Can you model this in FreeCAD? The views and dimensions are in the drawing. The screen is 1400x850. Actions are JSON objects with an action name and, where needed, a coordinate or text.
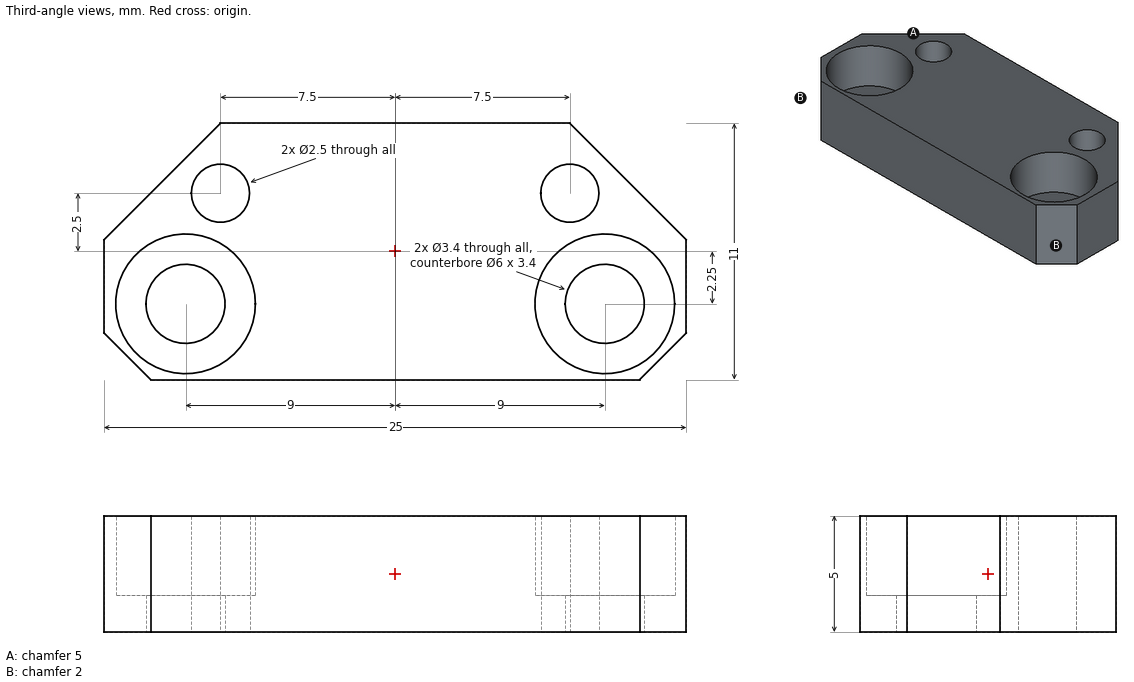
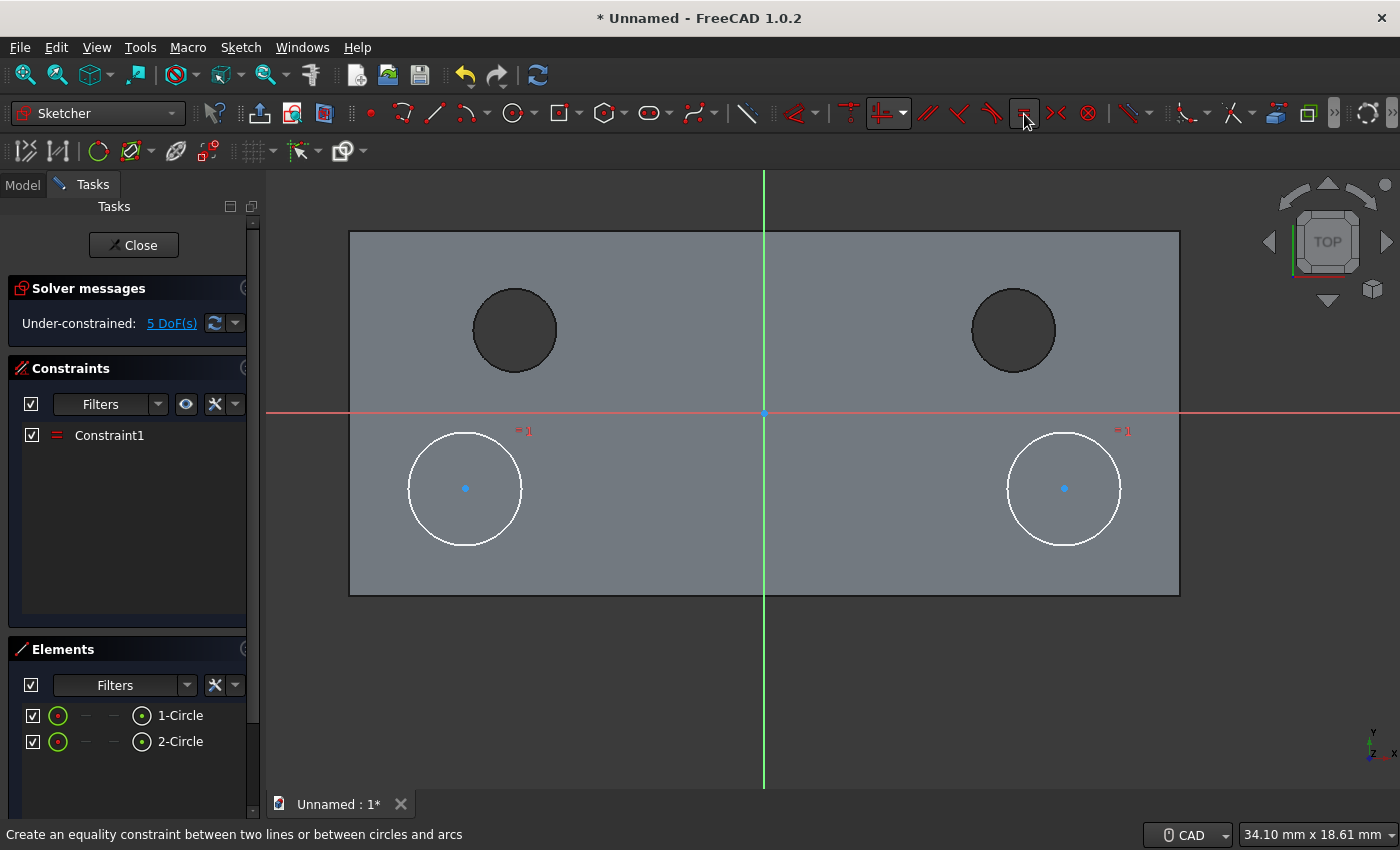
{"action": "left_click", "coordinate": [1064, 489]}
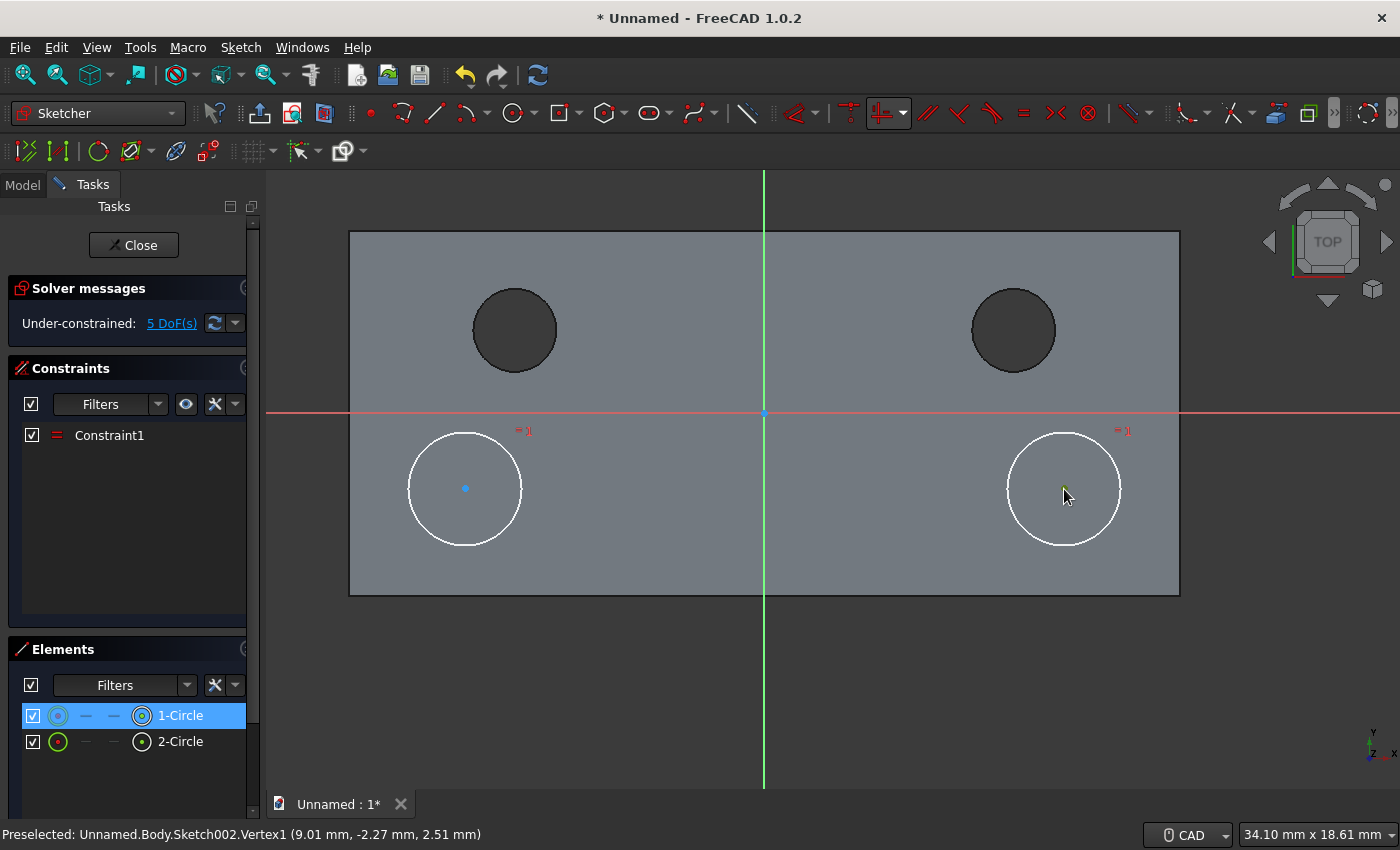
{"action": "left_click", "coordinate": [465, 489]}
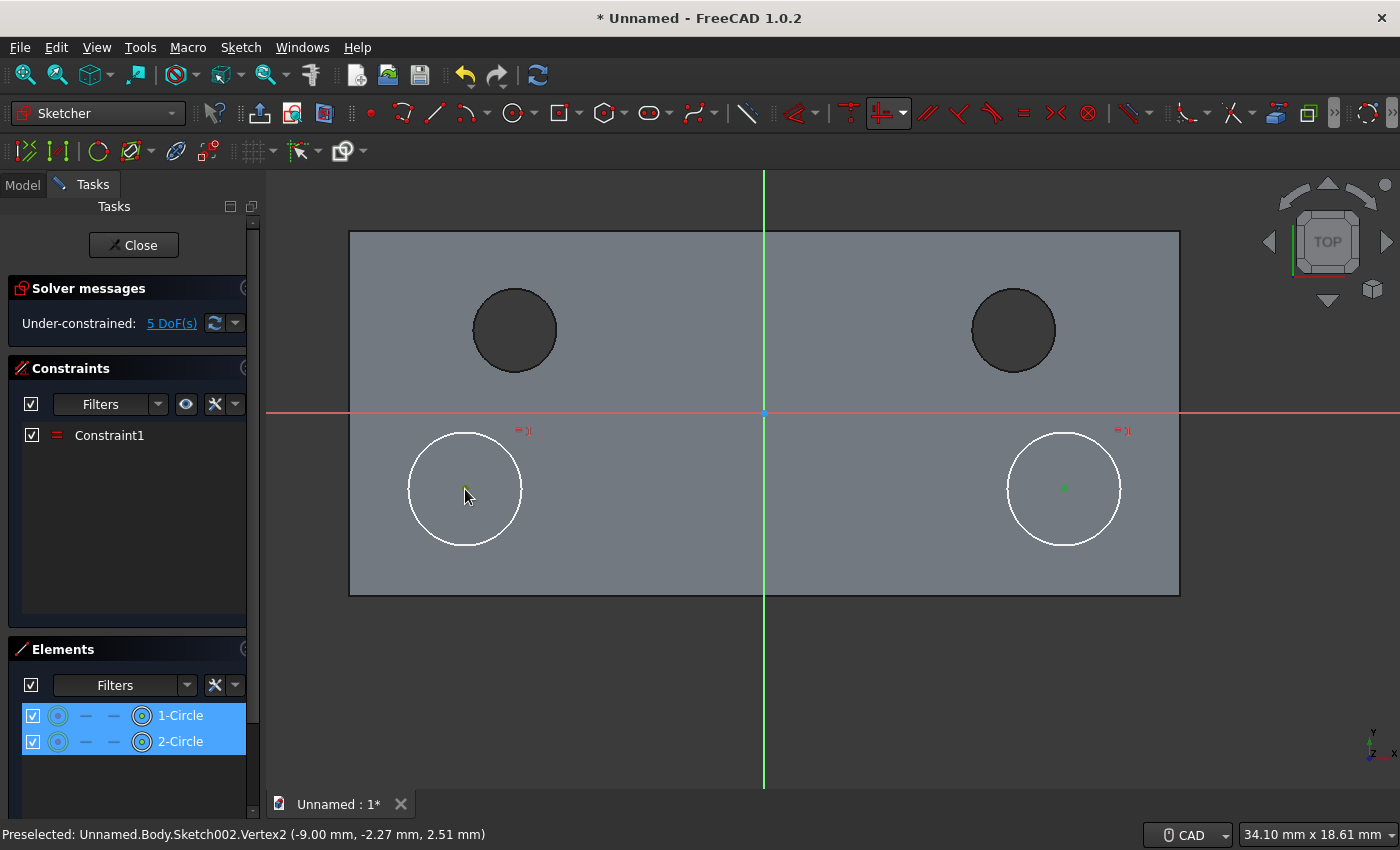
{"action": "key", "text": "h"}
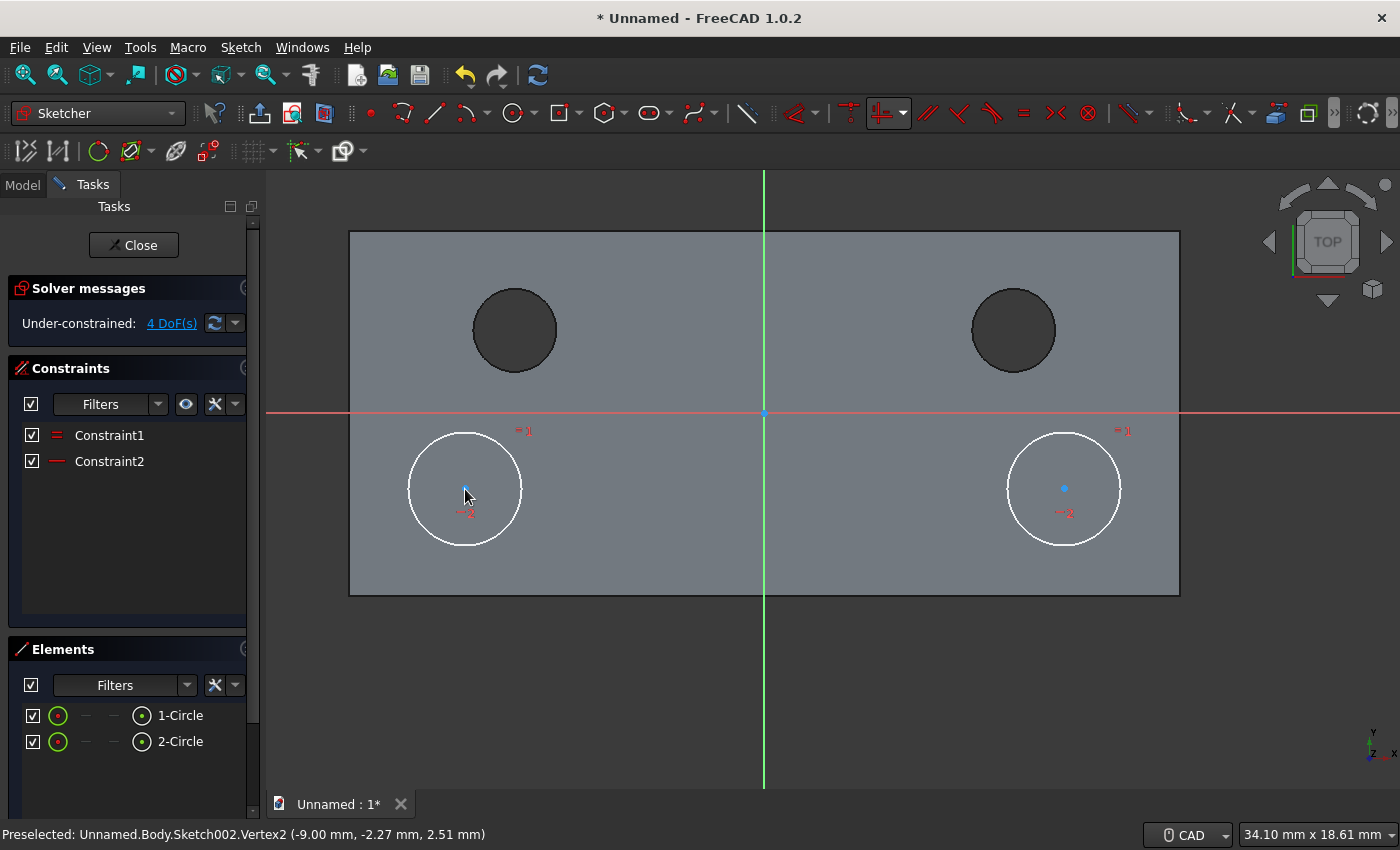
{"action": "key", "text": "d"}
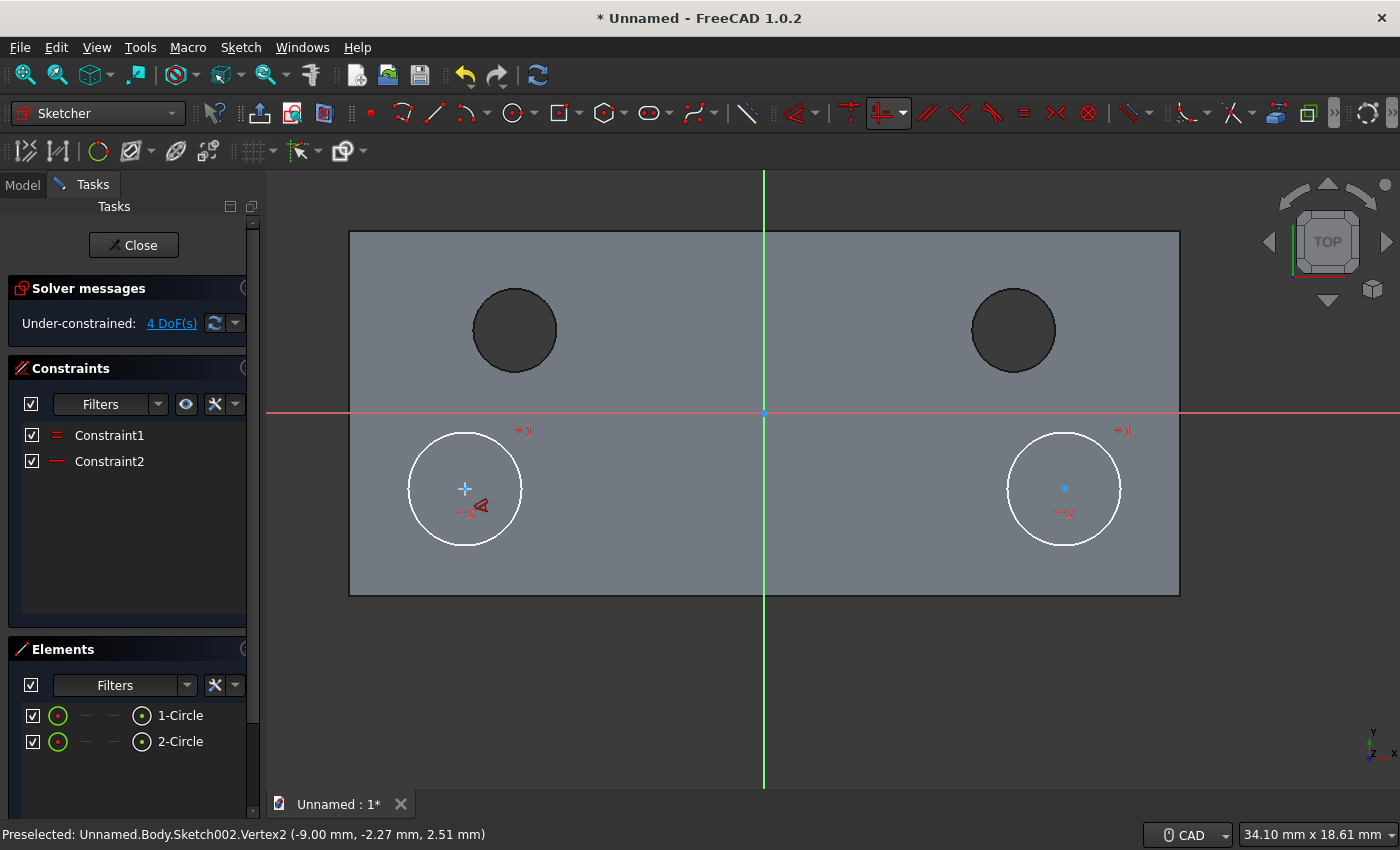
{"action": "left_click", "coordinate": [1104, 449]}
{"action": "left_click", "coordinate": [1149, 464]}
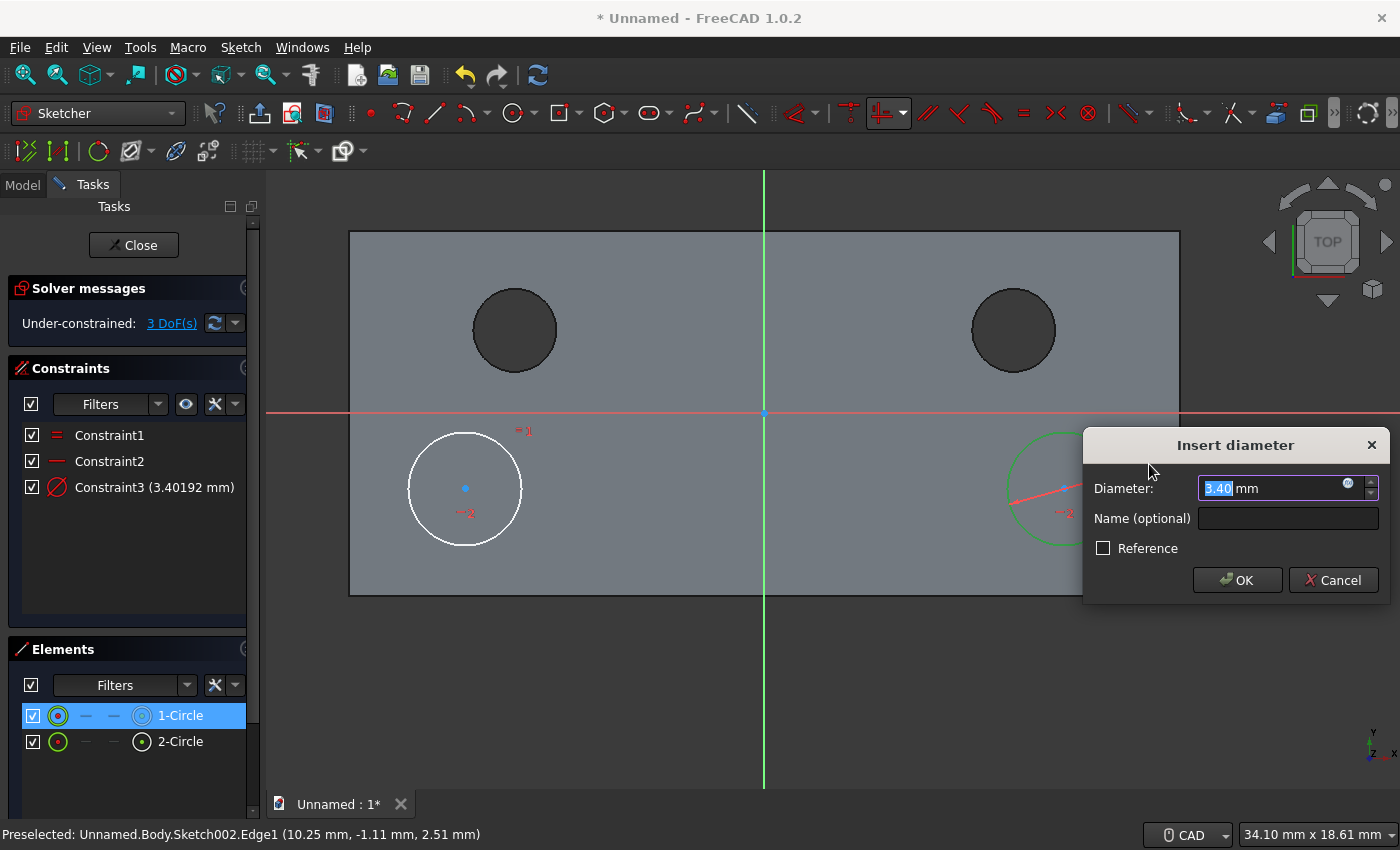
{"action": "type", "text": "3.4"}
{"action": "key", "text": "Return"}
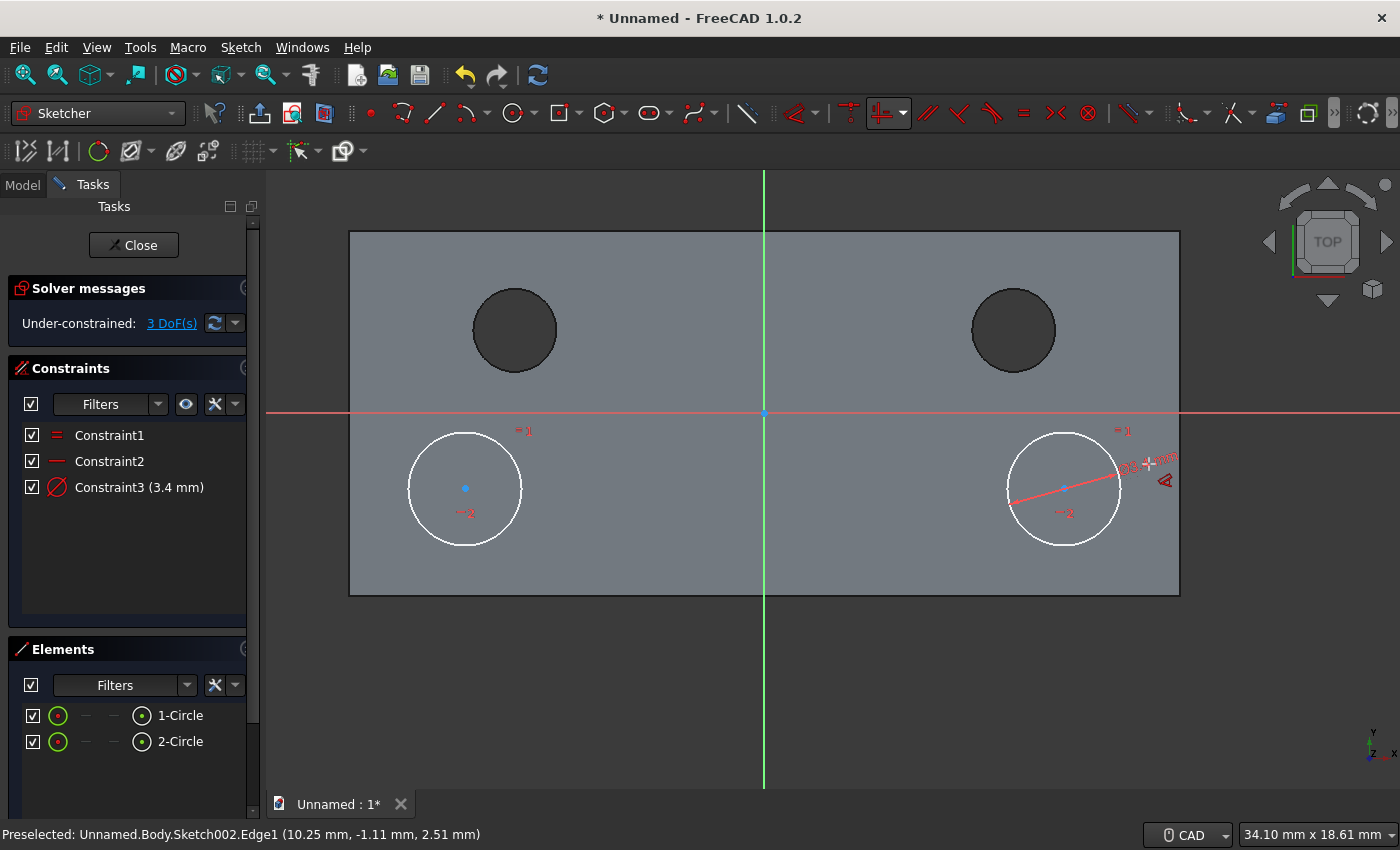
{"action": "left_click", "coordinate": [1064, 489]}
{"action": "left_click", "coordinate": [914, 379]}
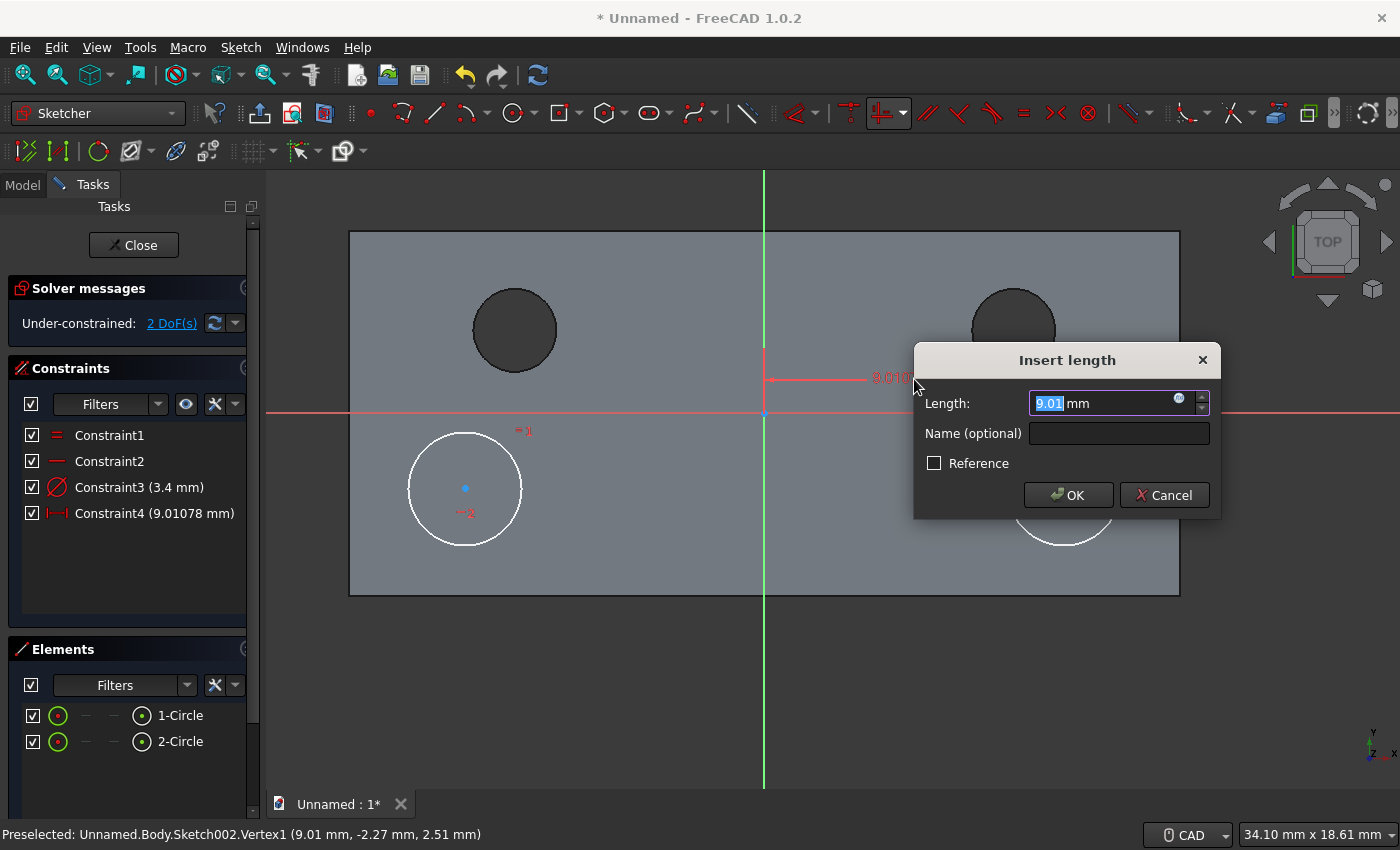
{"action": "type", "text": "9"}
{"action": "key", "text": "Return"}